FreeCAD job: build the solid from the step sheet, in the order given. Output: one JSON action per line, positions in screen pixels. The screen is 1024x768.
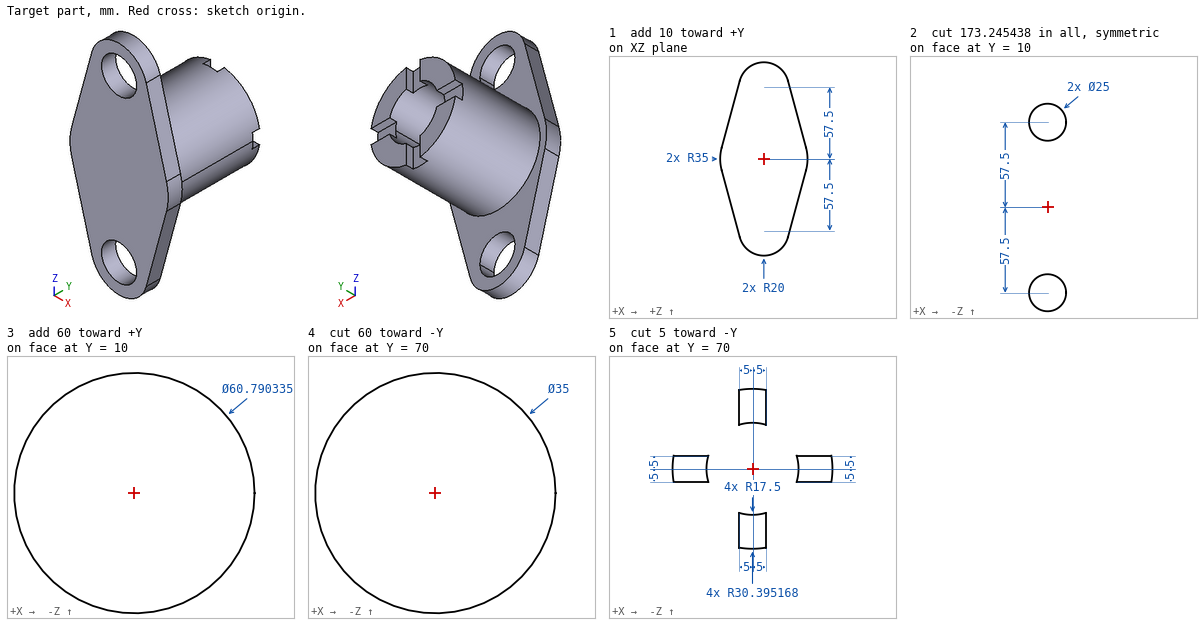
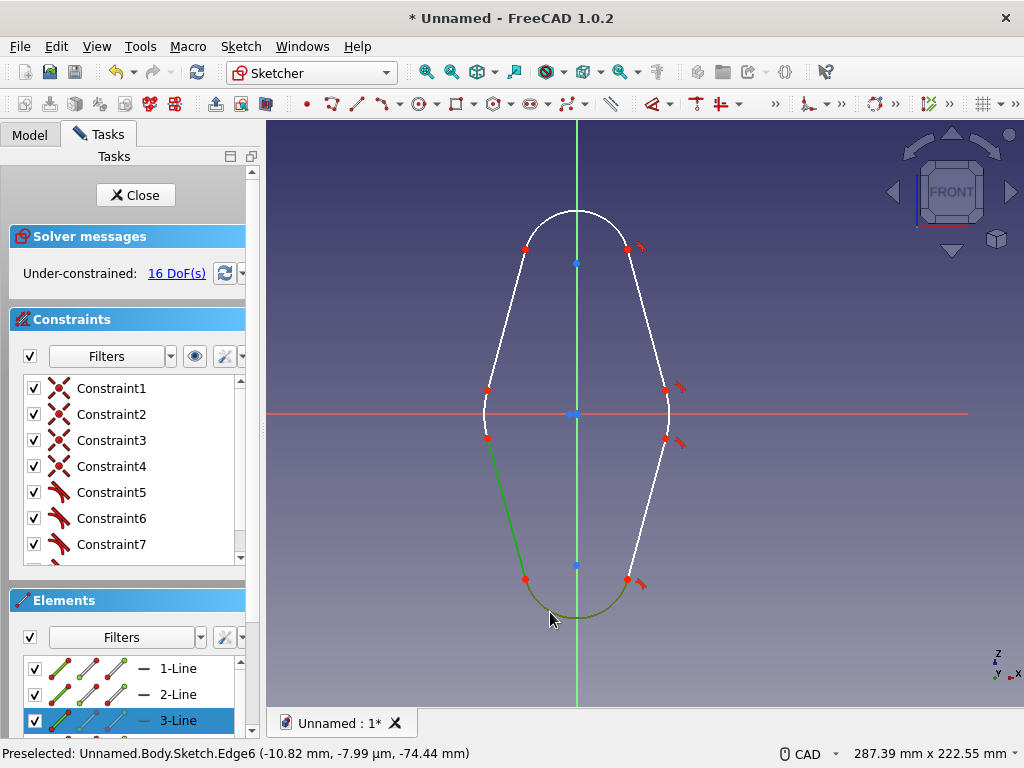
{"action": "key", "text": "t"}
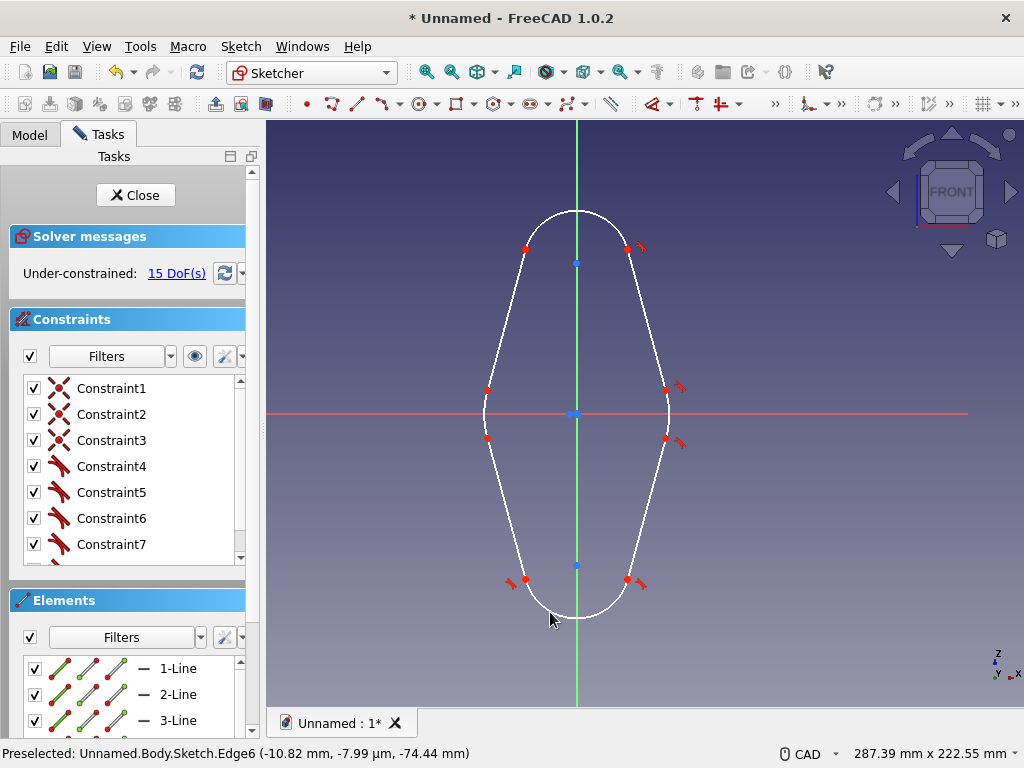
{"action": "left_click", "coordinate": [514, 537]}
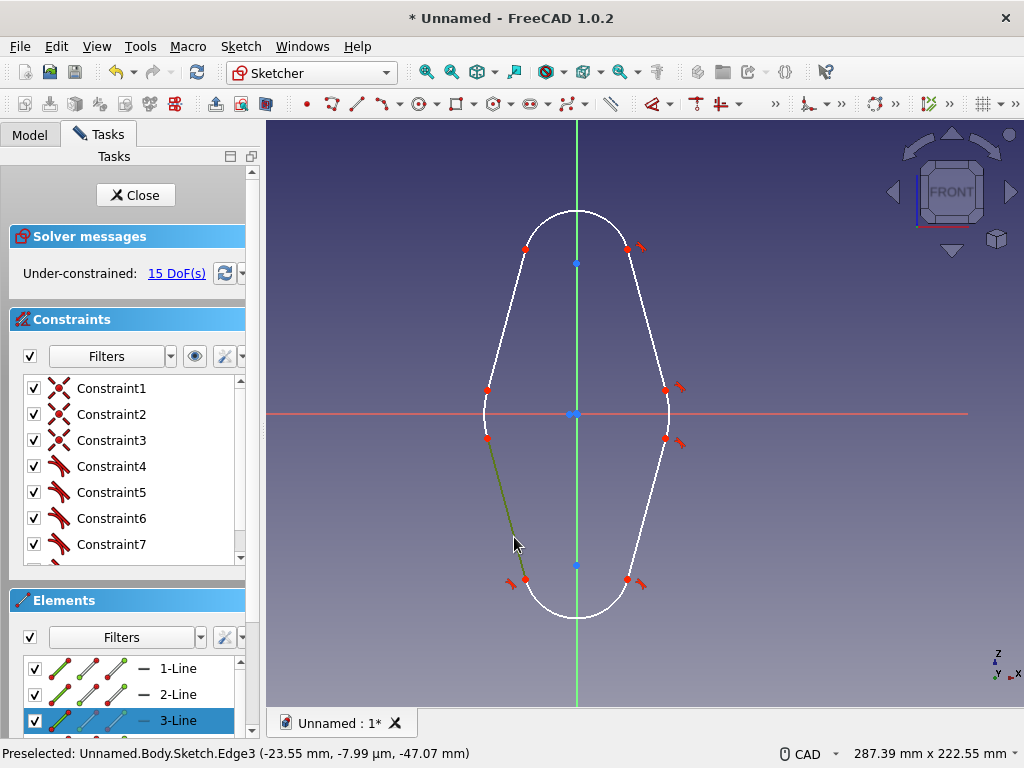
{"action": "scroll", "coordinate": [485, 424], "scroll_direction": "up", "scroll_amount": 2}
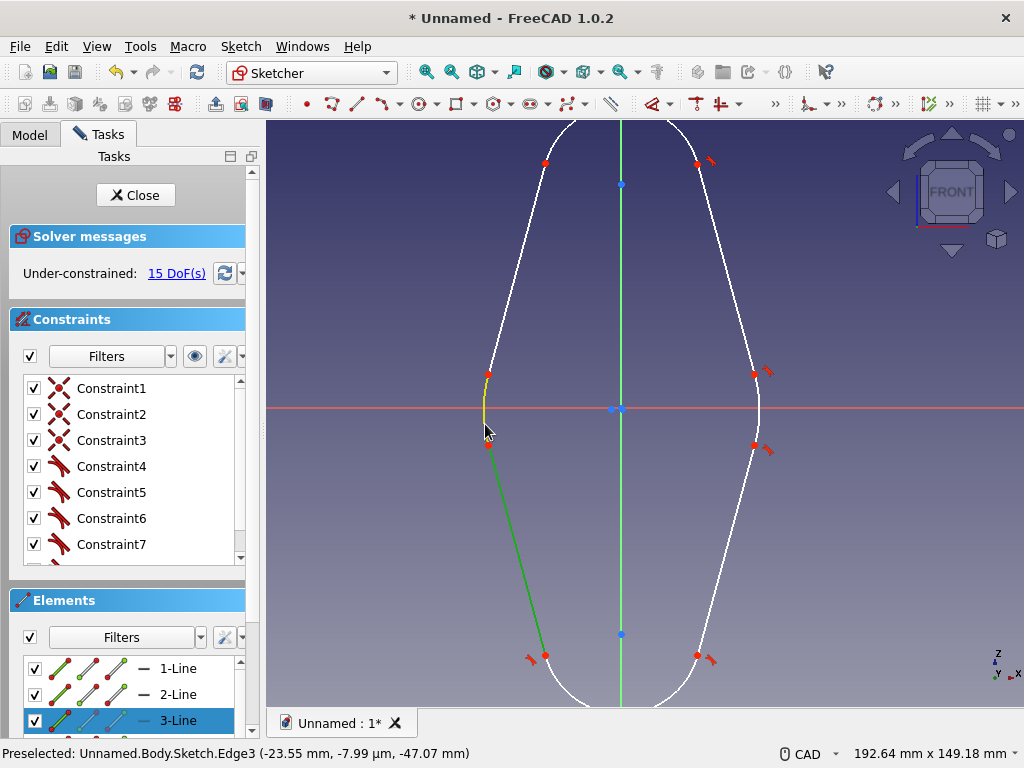
{"action": "left_click", "coordinate": [485, 424]}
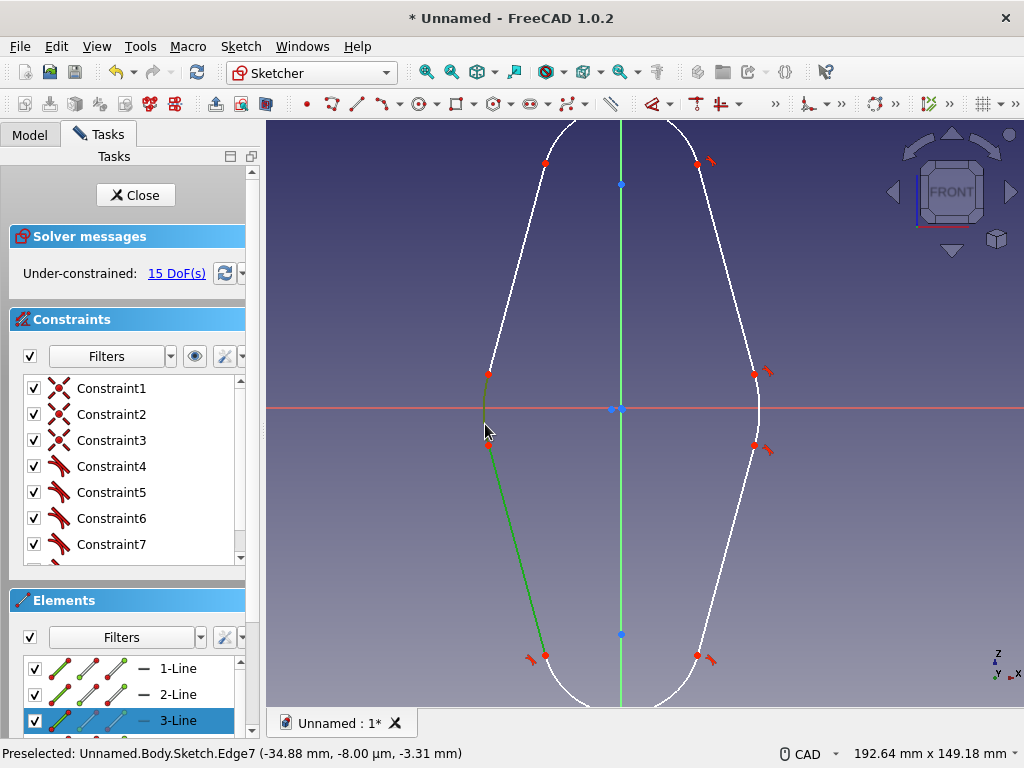
{"action": "key", "text": "t"}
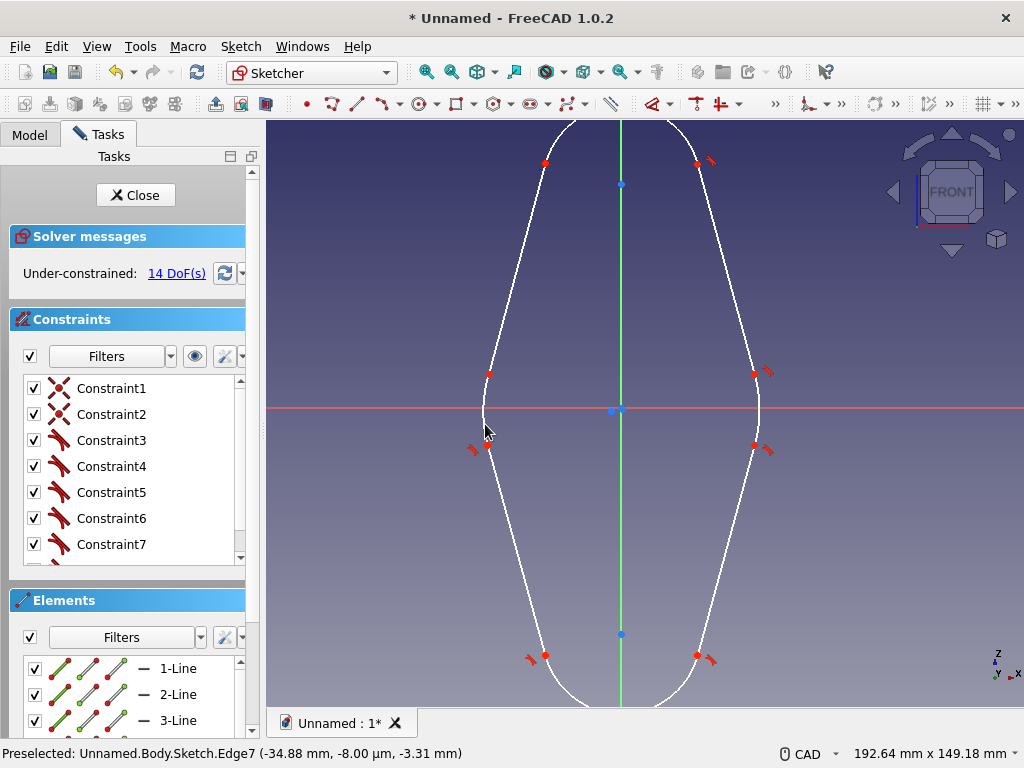
{"action": "left_click", "coordinate": [506, 311]}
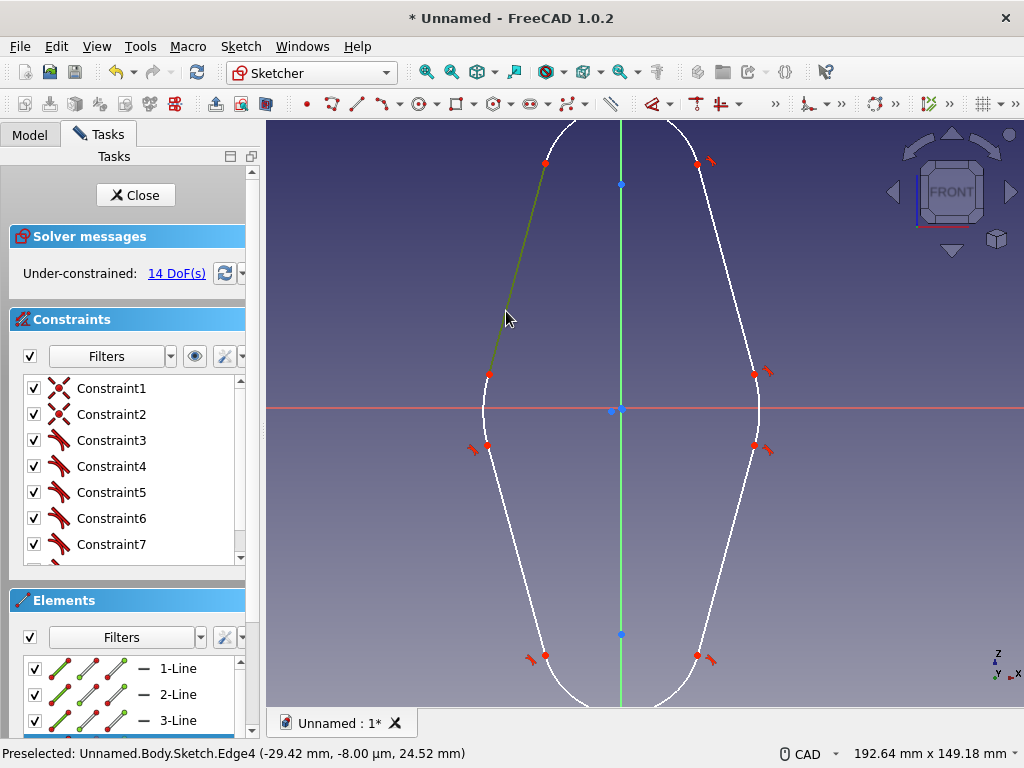
{"action": "left_click", "coordinate": [484, 395]}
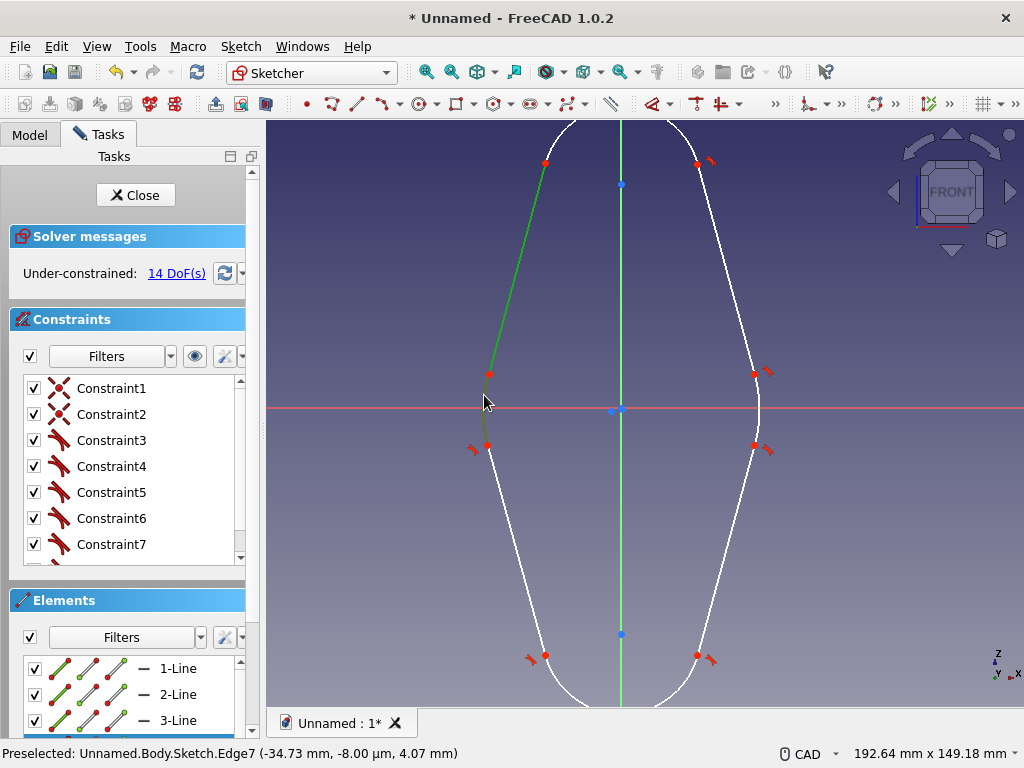
{"action": "key", "text": "t"}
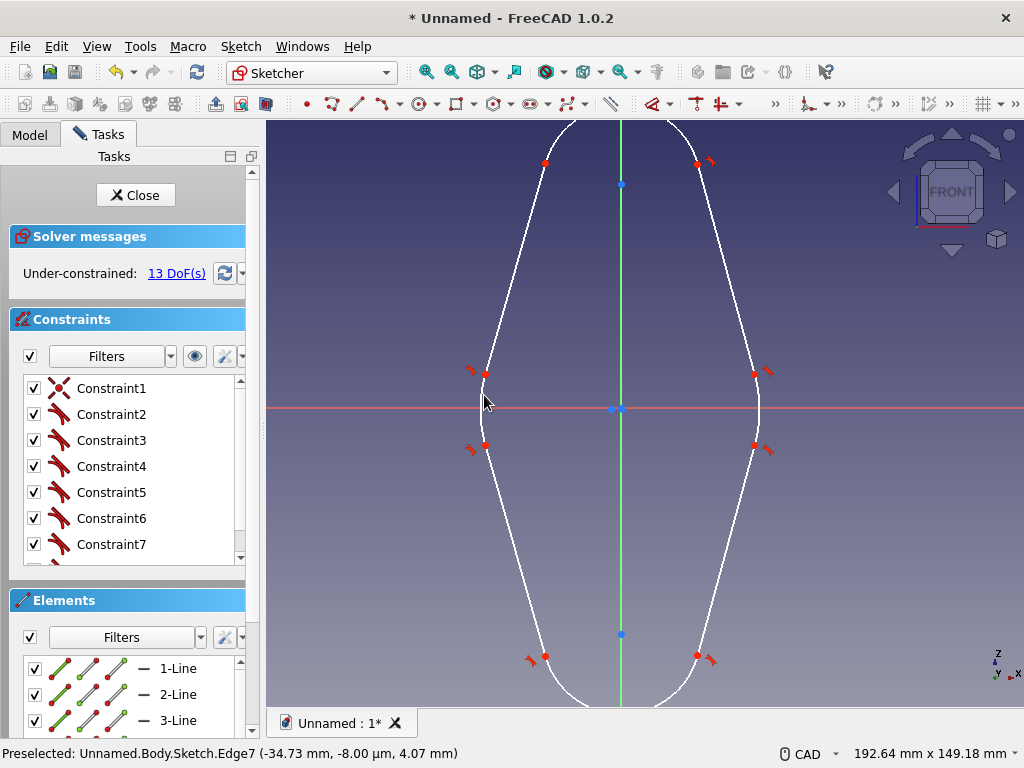
{"action": "left_click", "coordinate": [504, 311]}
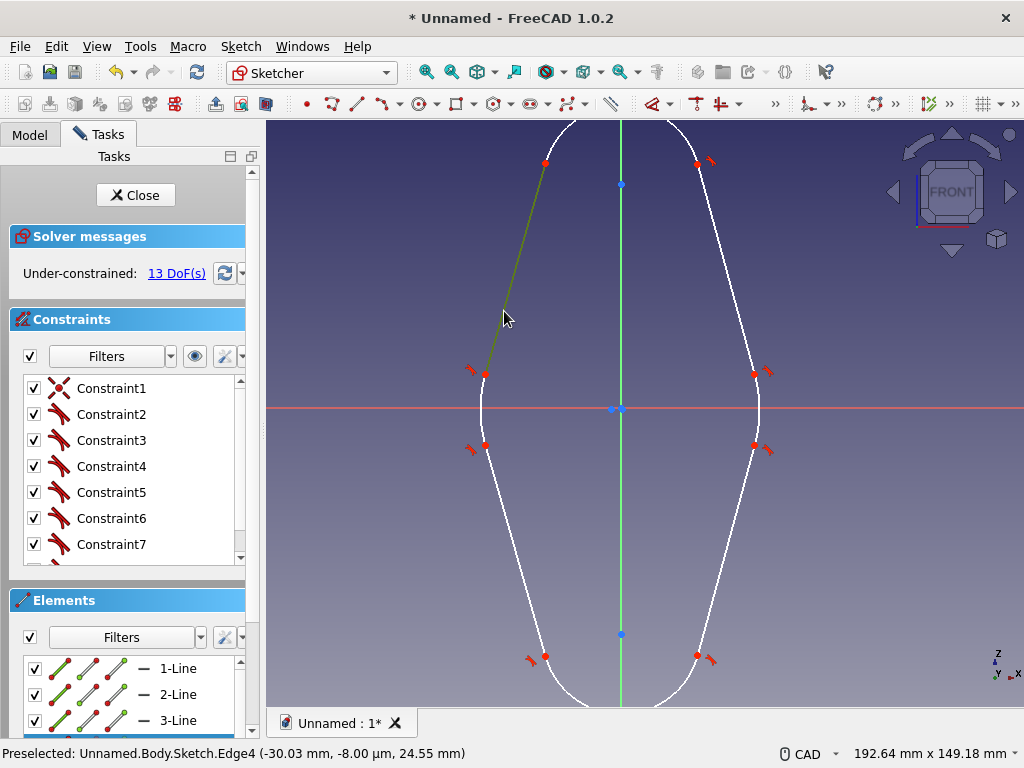
{"action": "scroll", "coordinate": [485, 424], "scroll_direction": "down", "scroll_amount": 2}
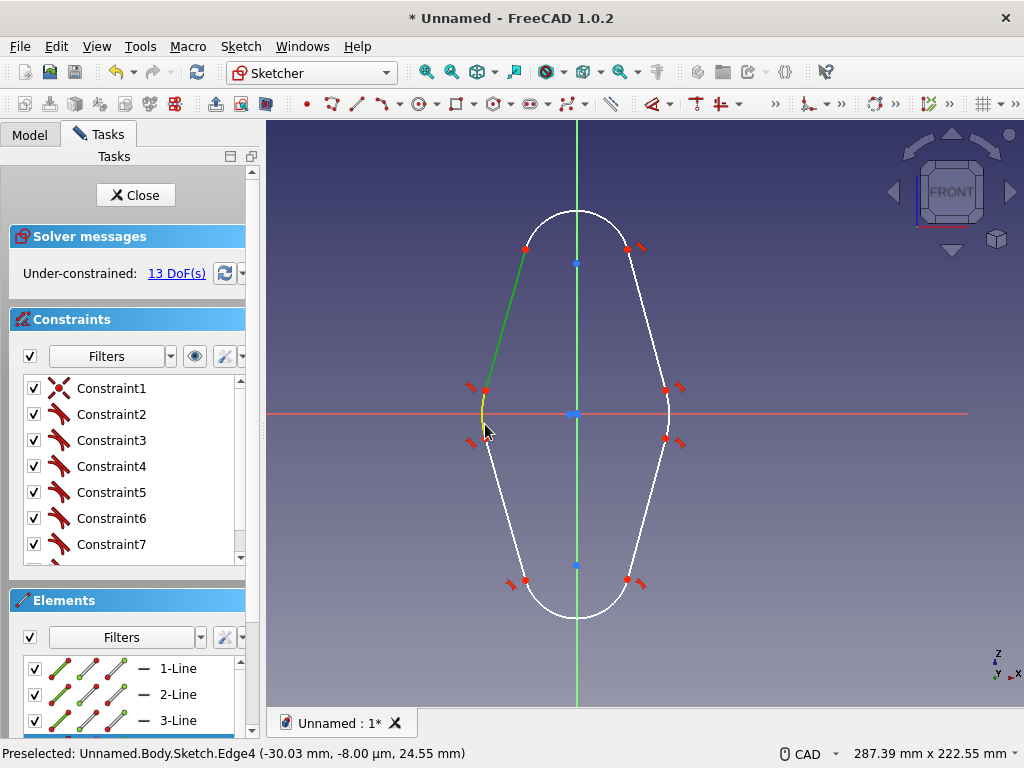
{"action": "left_click", "coordinate": [603, 218]}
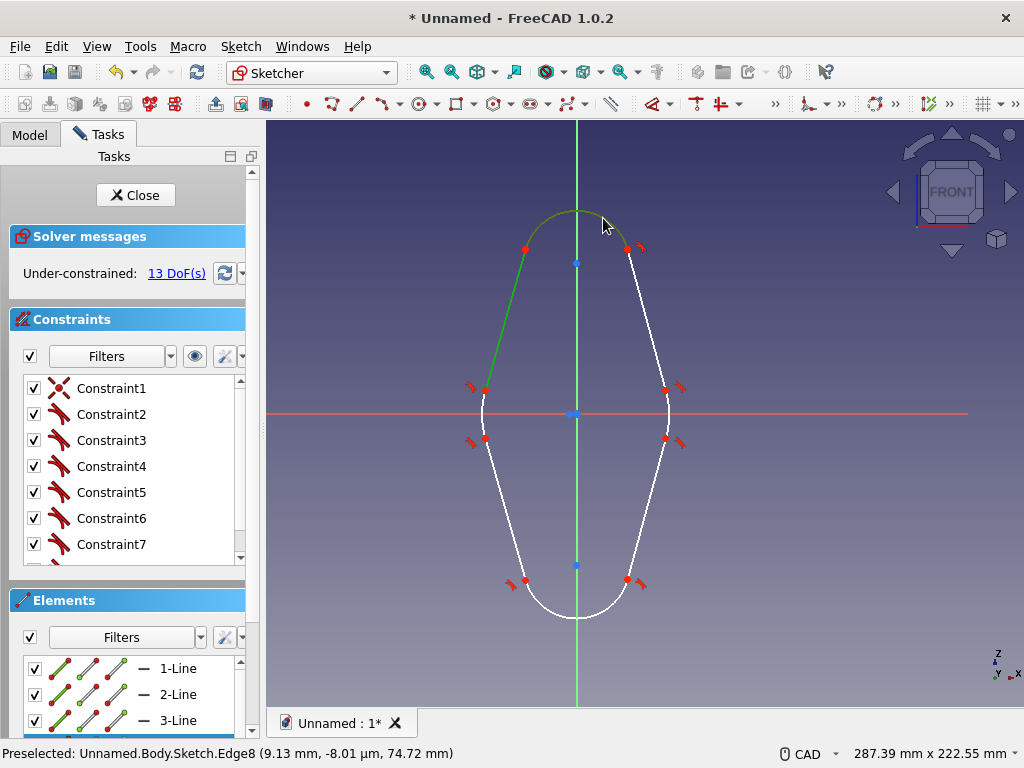
{"action": "key", "text": "t"}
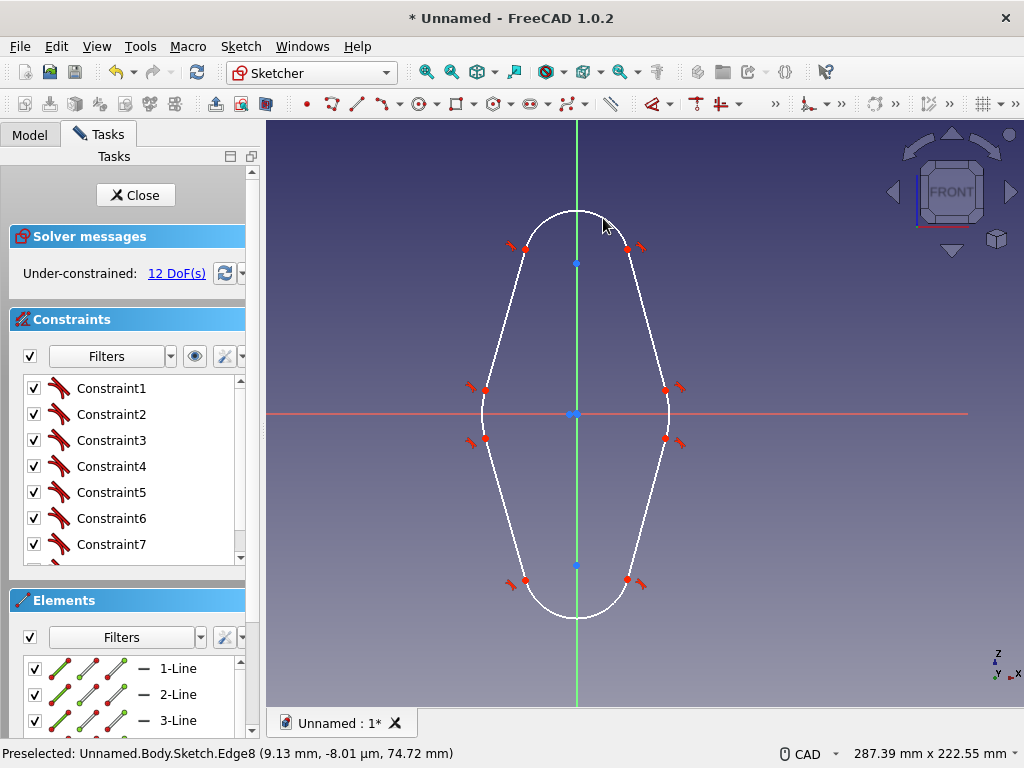
{"action": "scroll", "coordinate": [669, 424], "scroll_direction": "up", "scroll_amount": 2}